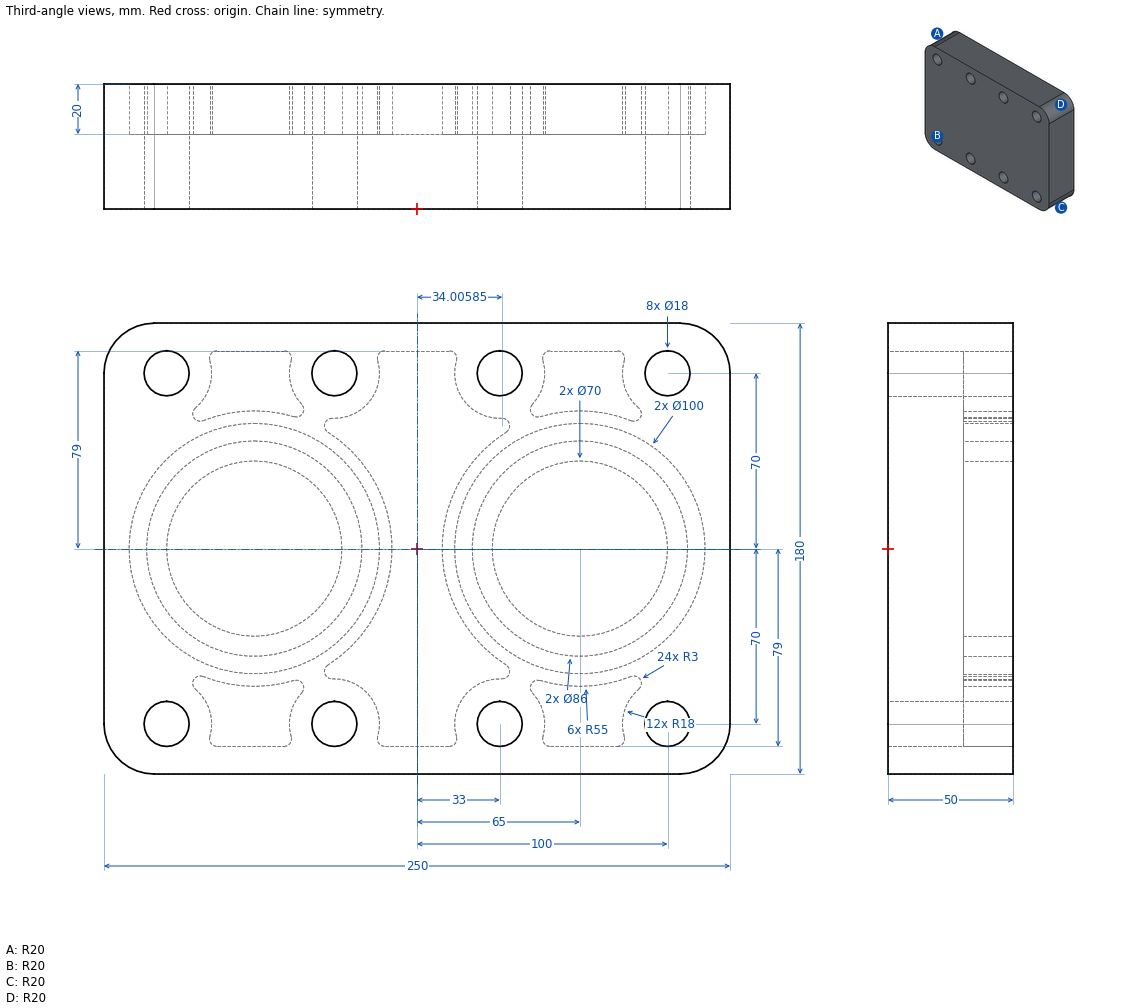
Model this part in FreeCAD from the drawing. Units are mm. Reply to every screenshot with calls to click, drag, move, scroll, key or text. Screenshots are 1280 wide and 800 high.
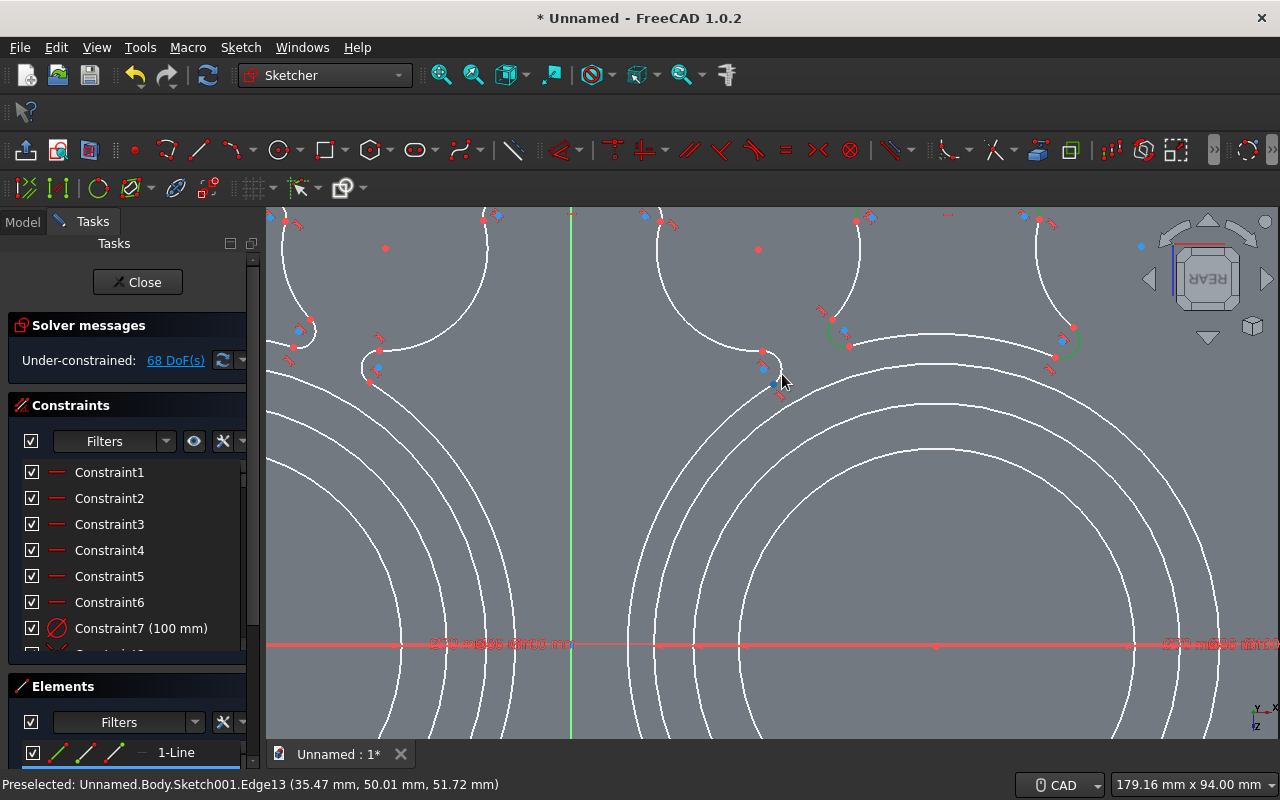
click(781, 373)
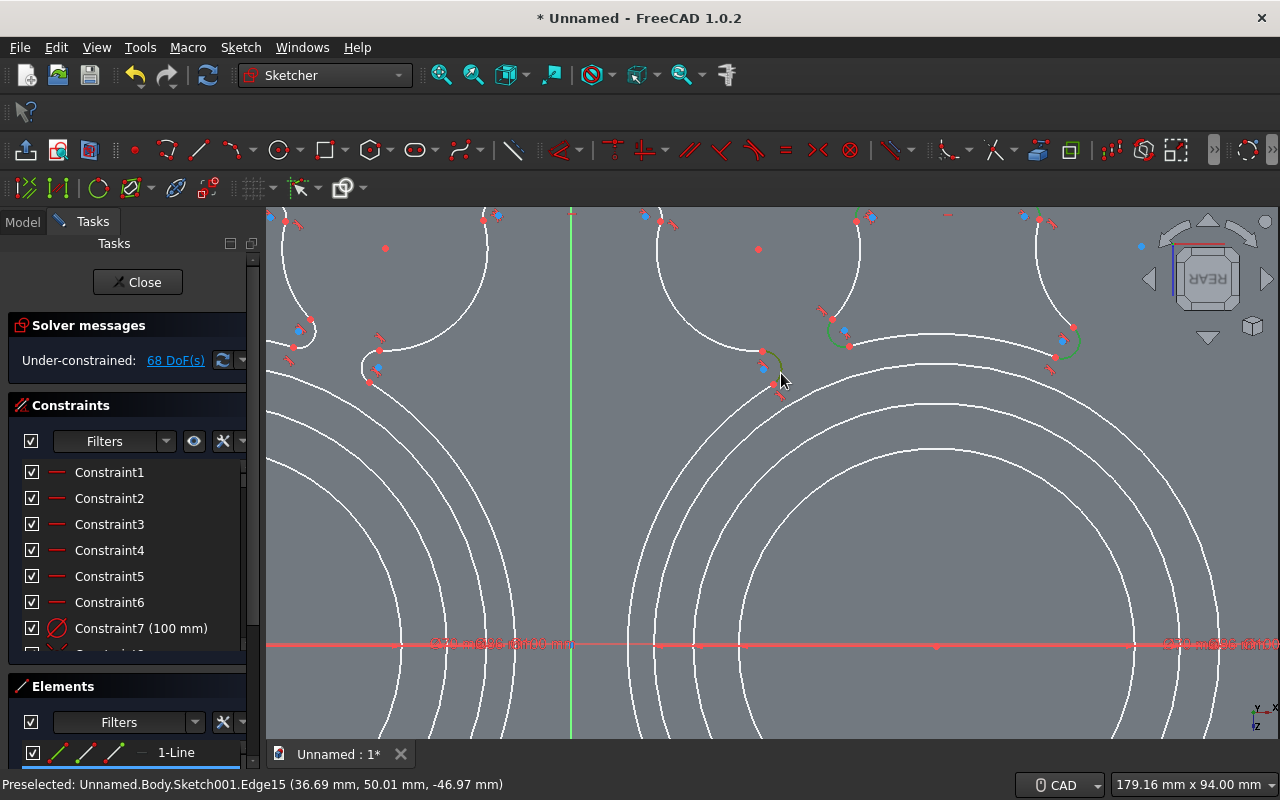
scroll(782, 373, down, 5)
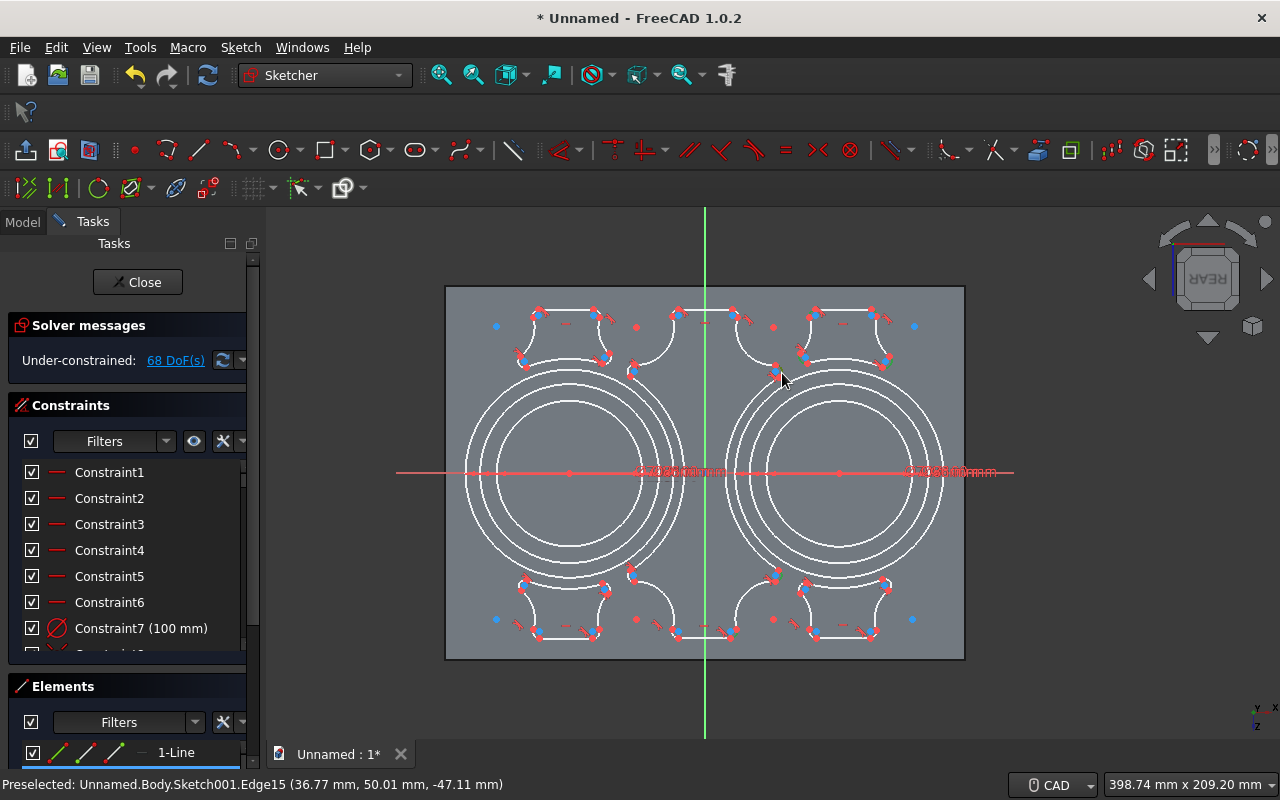
scroll(738, 314, up, 8)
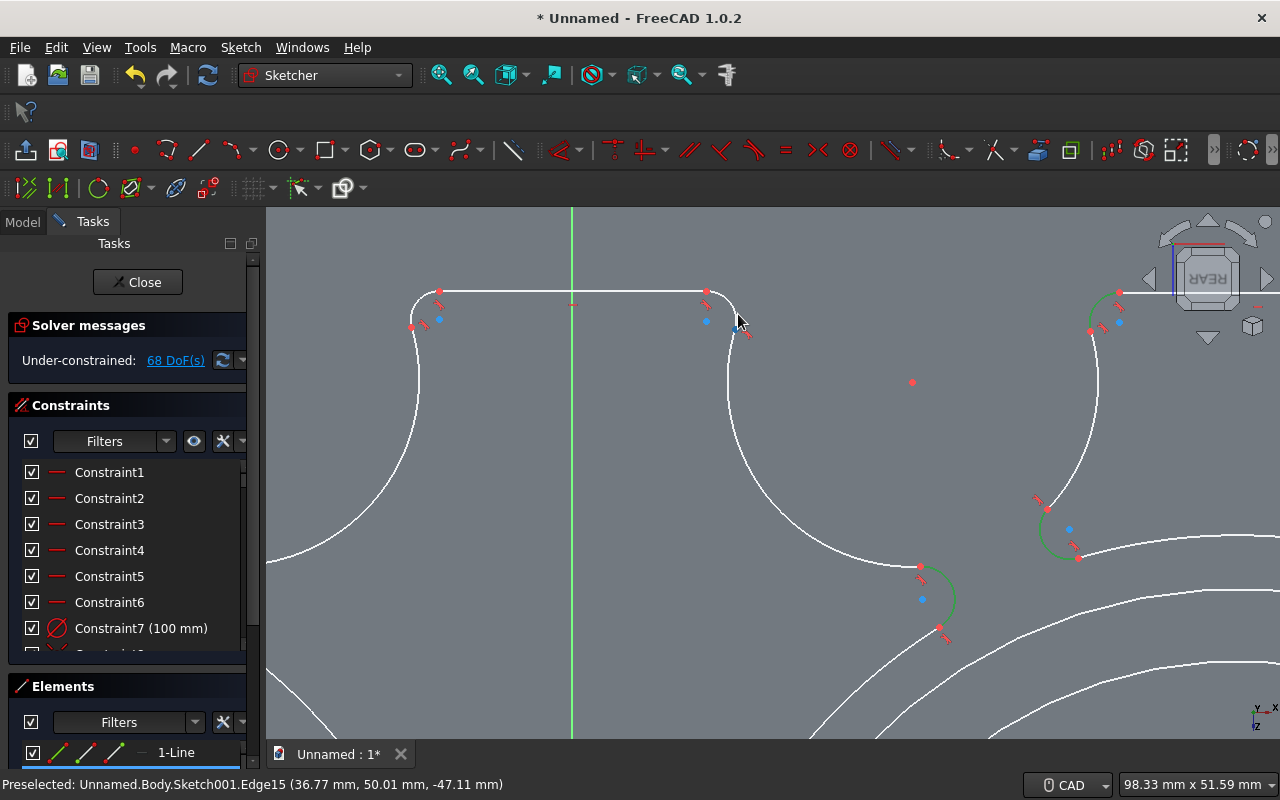
click(735, 313)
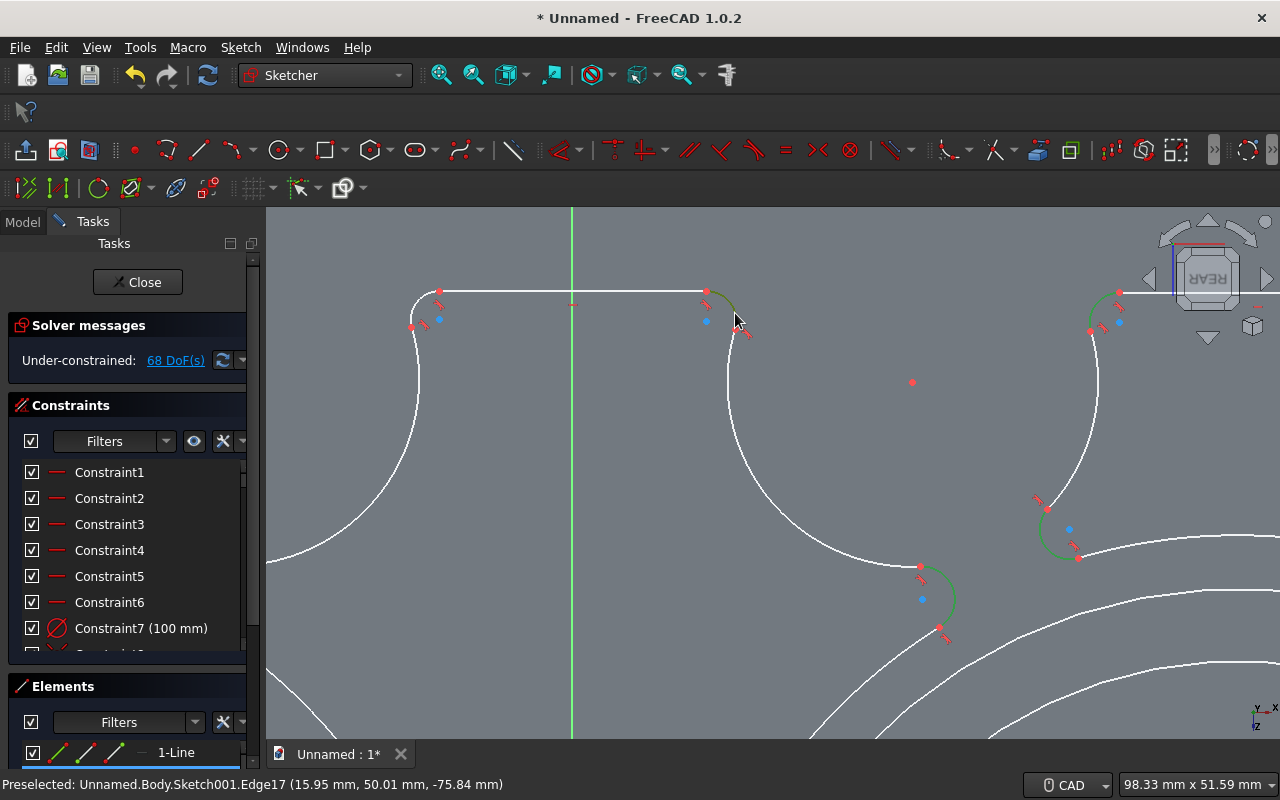
click(424, 296)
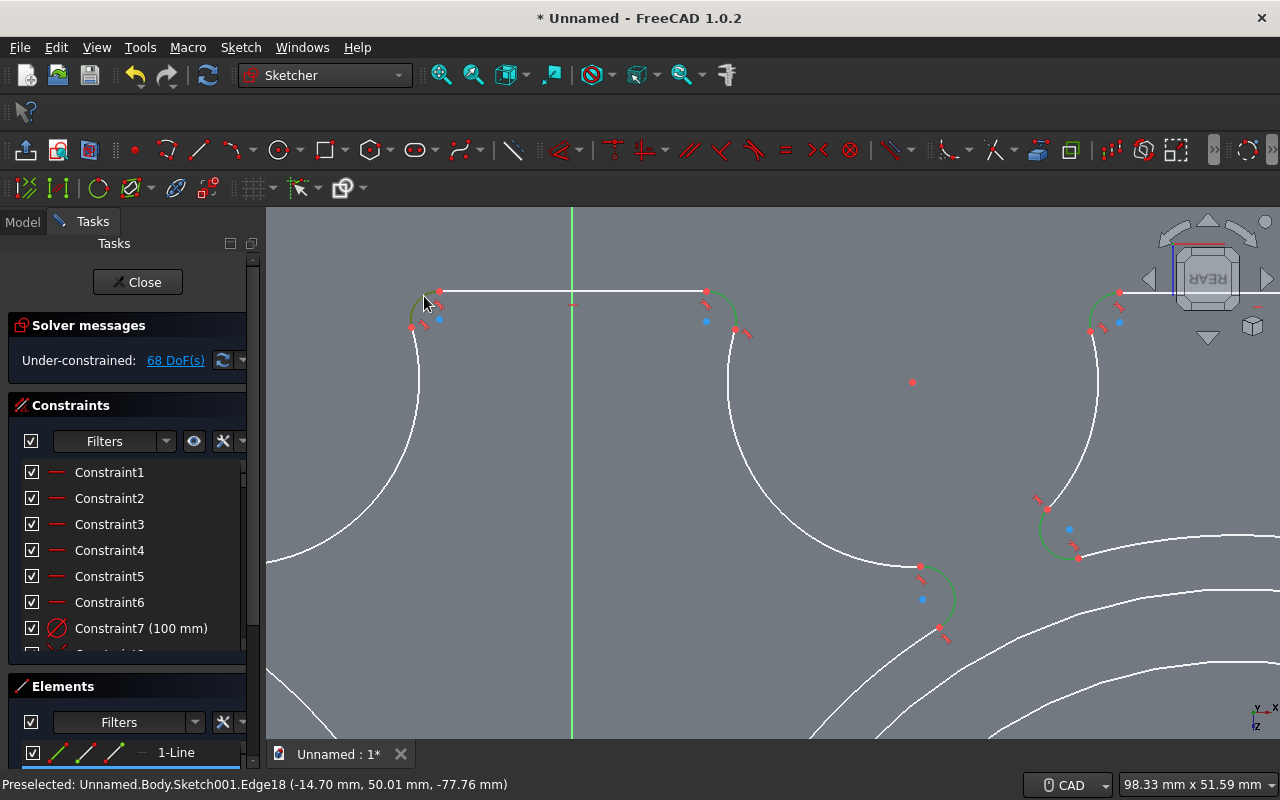
scroll(738, 314, down, 8)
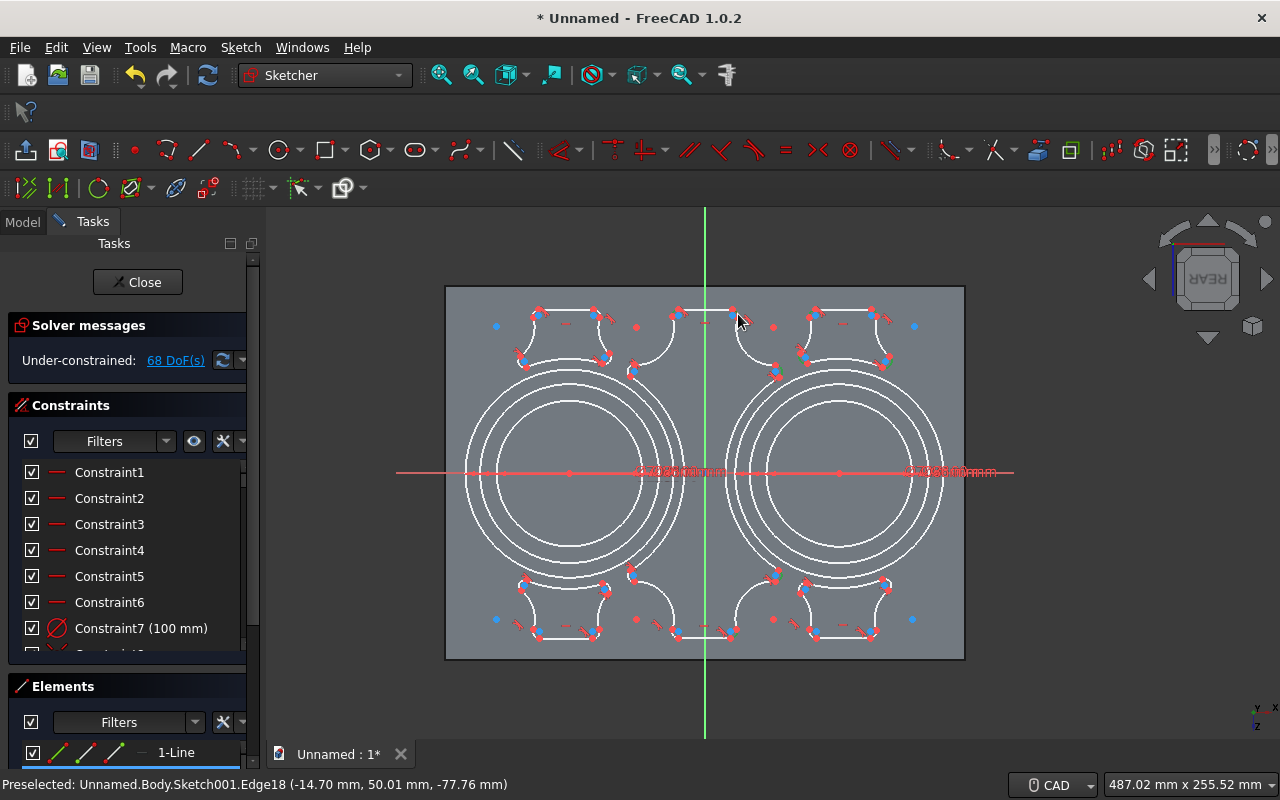
scroll(630, 367, up, 6)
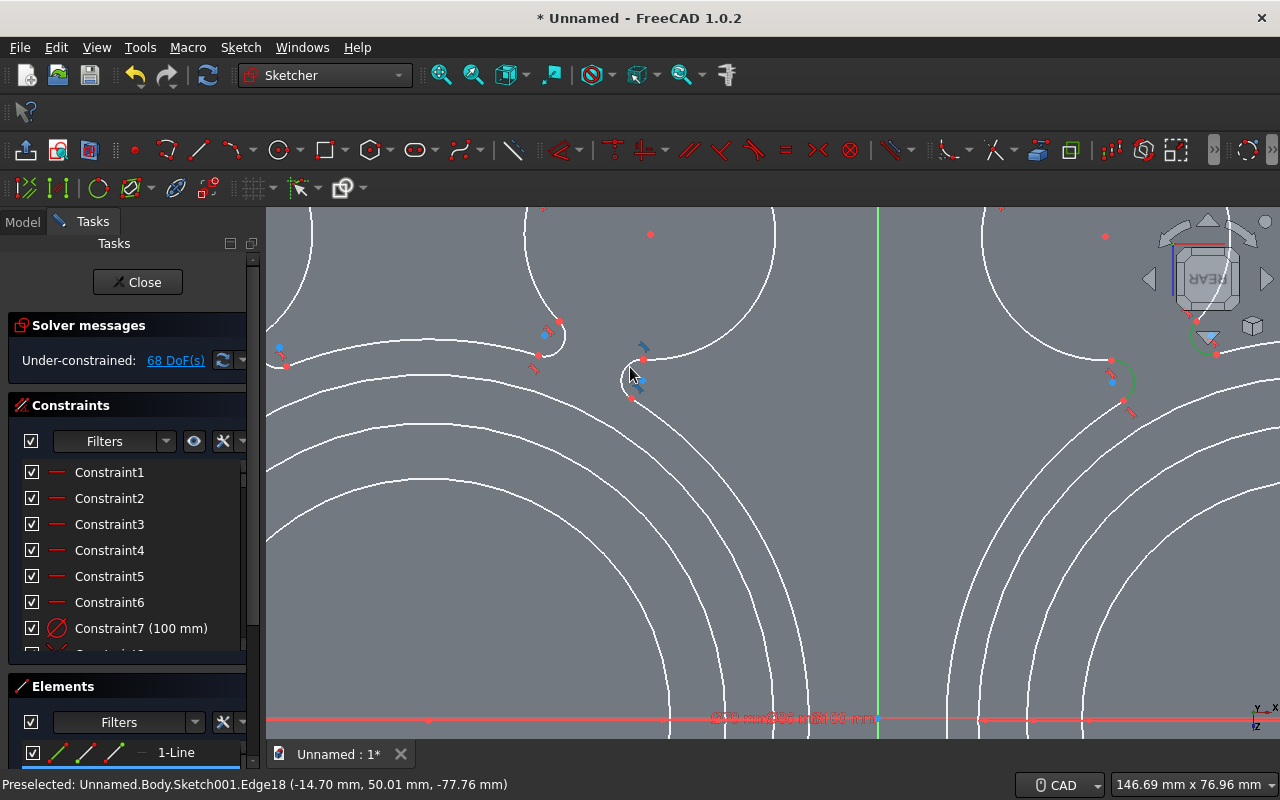
click(628, 365)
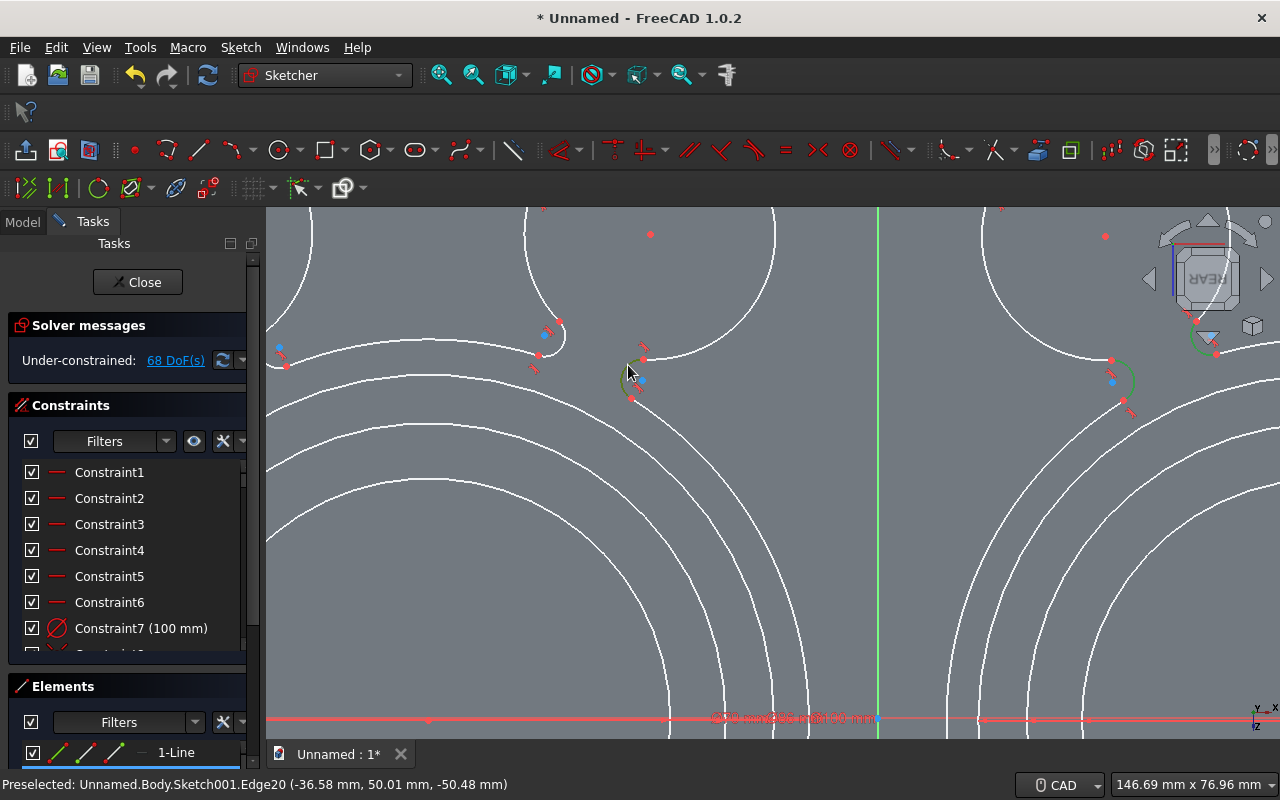
scroll(630, 367, down, 6)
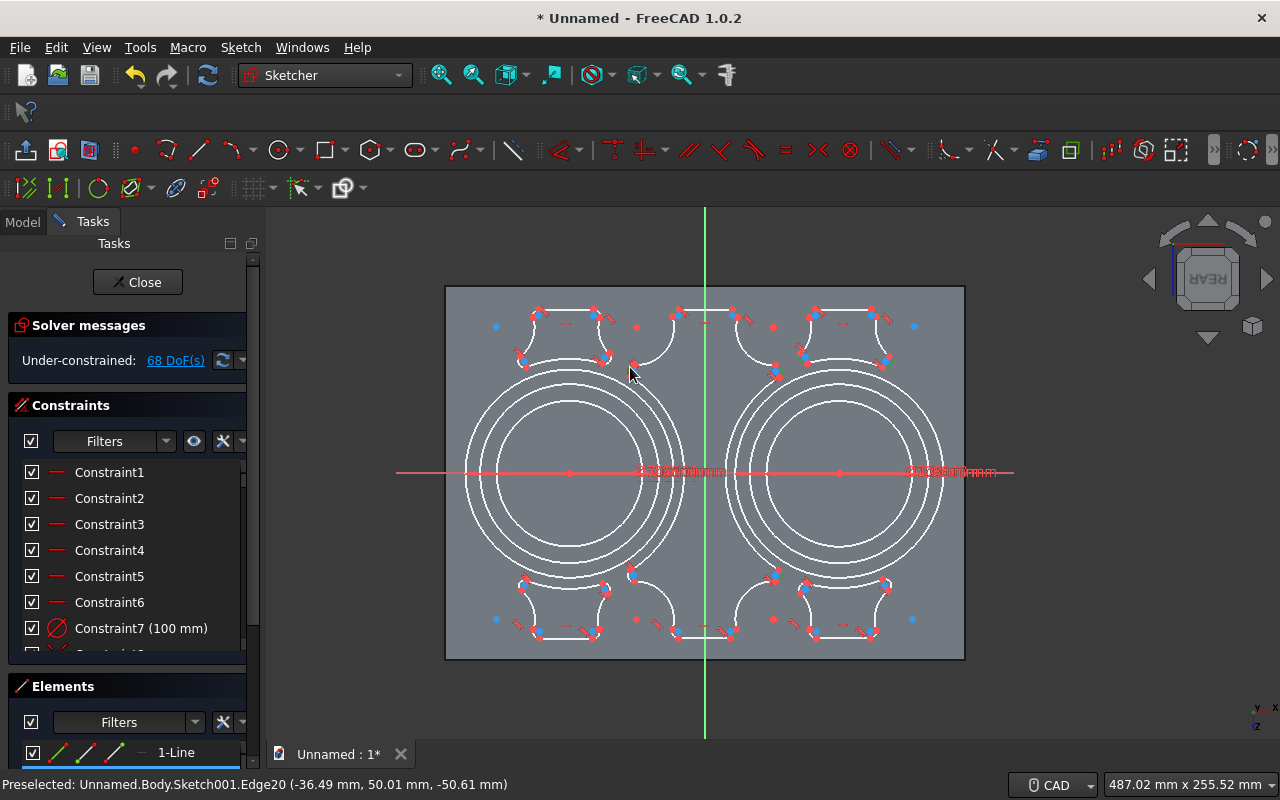
scroll(628, 574, up, 6)